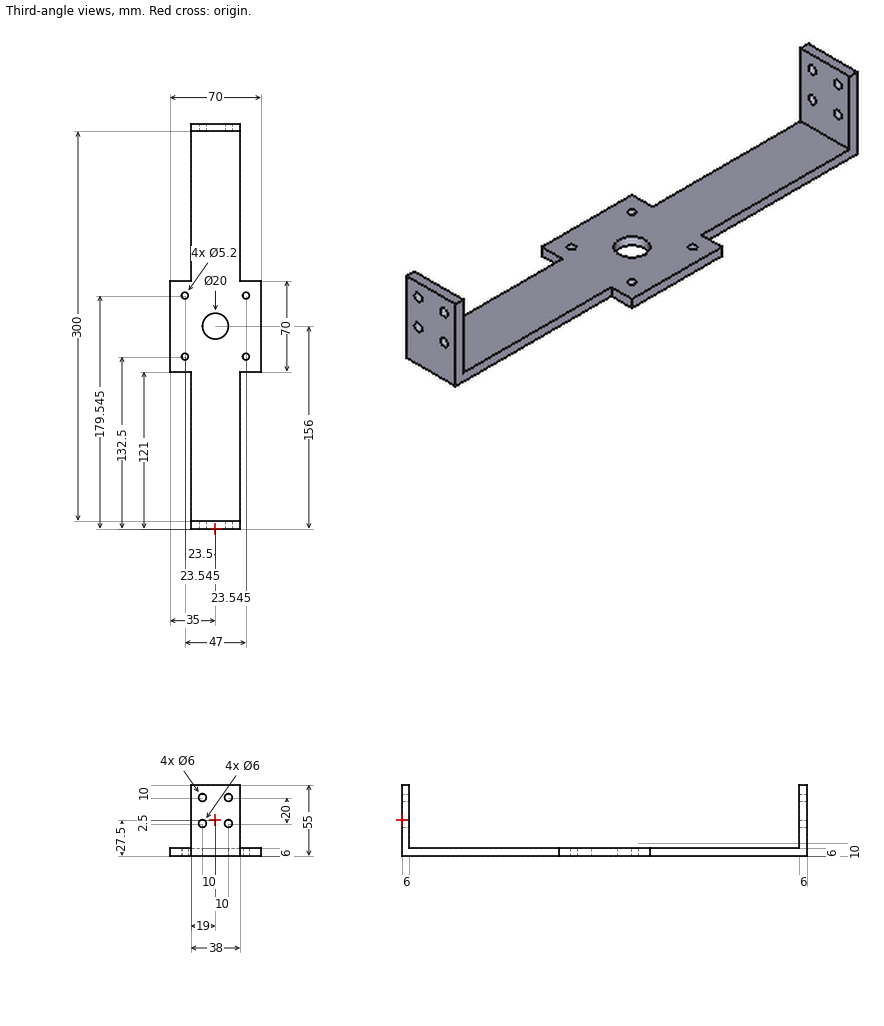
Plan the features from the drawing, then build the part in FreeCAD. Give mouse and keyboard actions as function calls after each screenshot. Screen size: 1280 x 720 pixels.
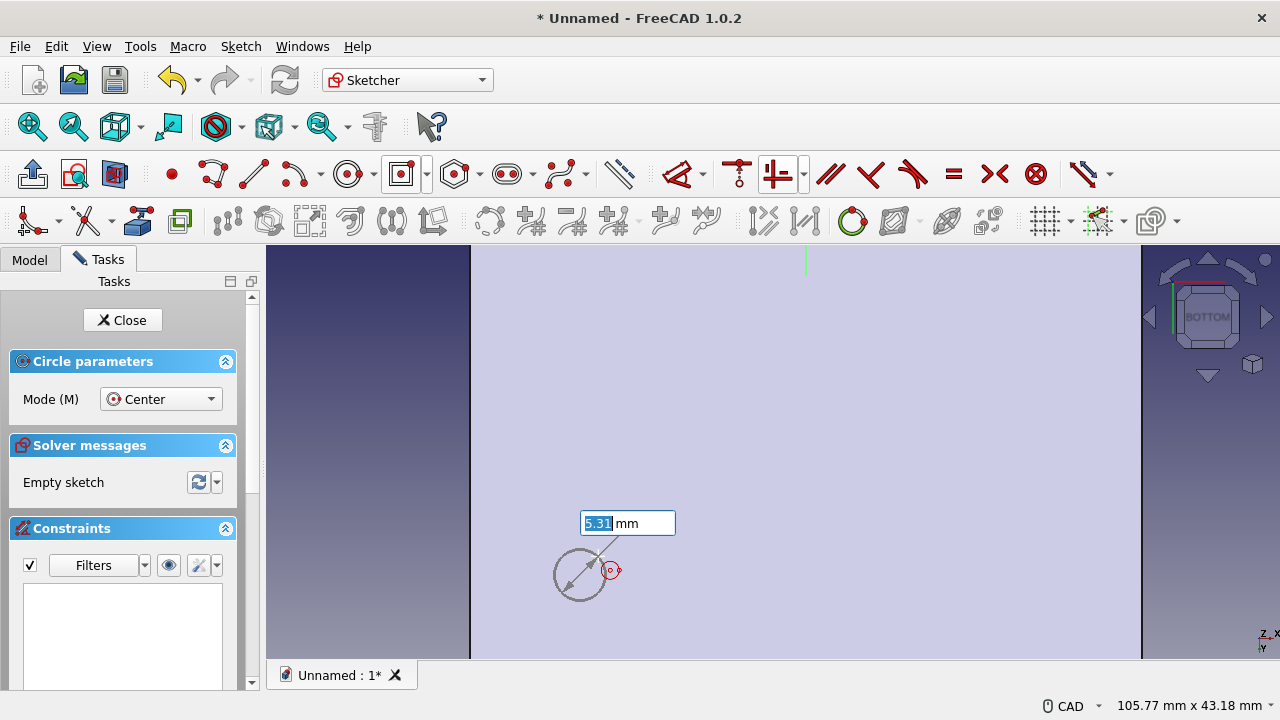
text(5.2)
key(Return)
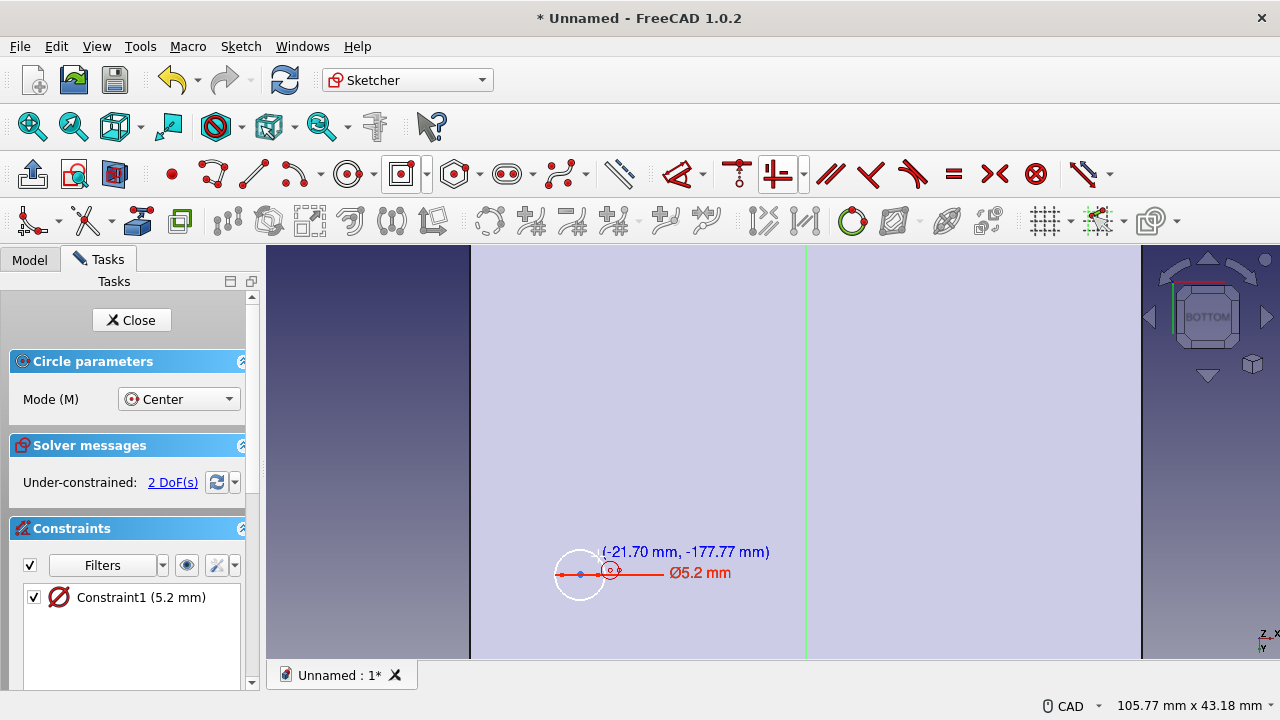
scroll(581, 578, down, 3)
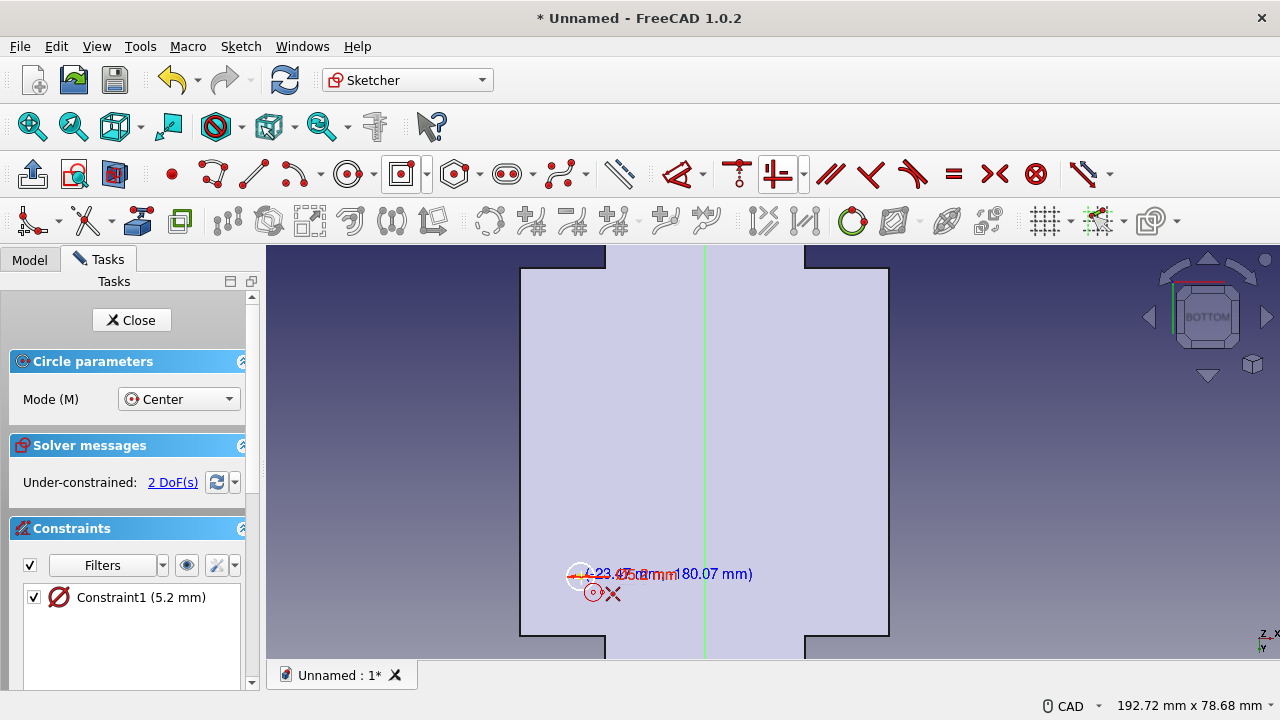
scroll(581, 329, up, 3)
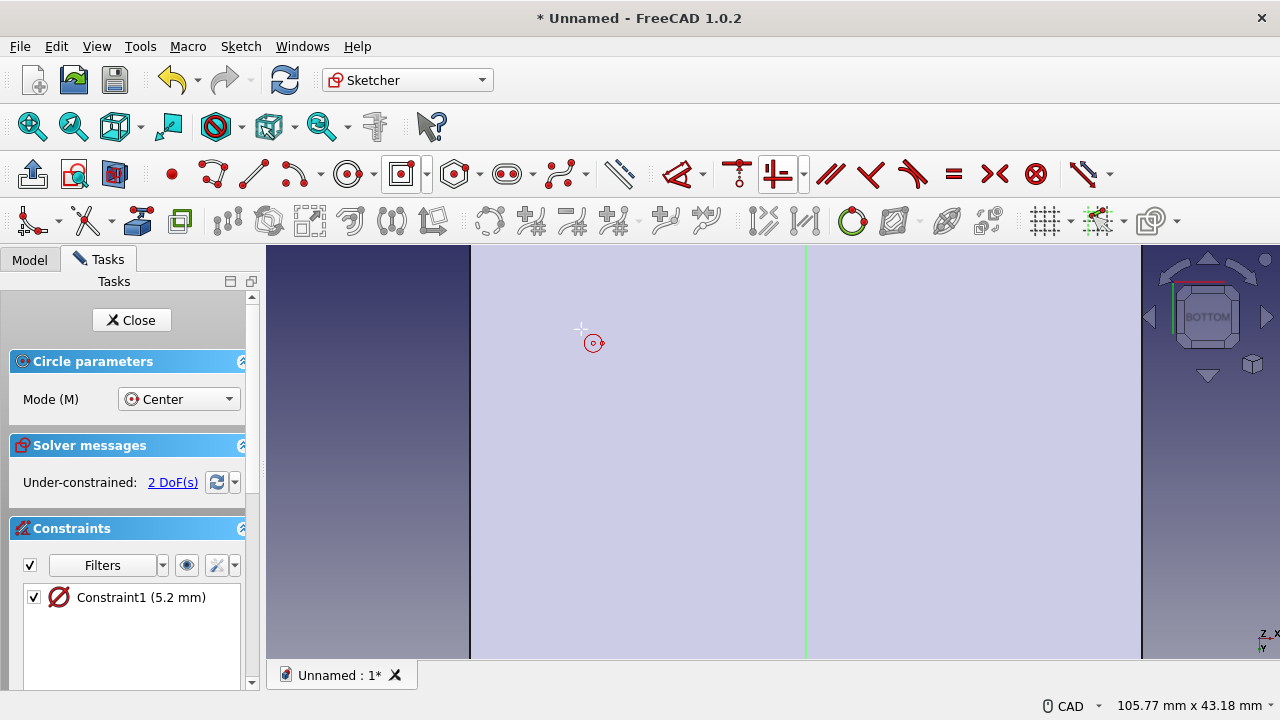
click(581, 328)
move(598, 311)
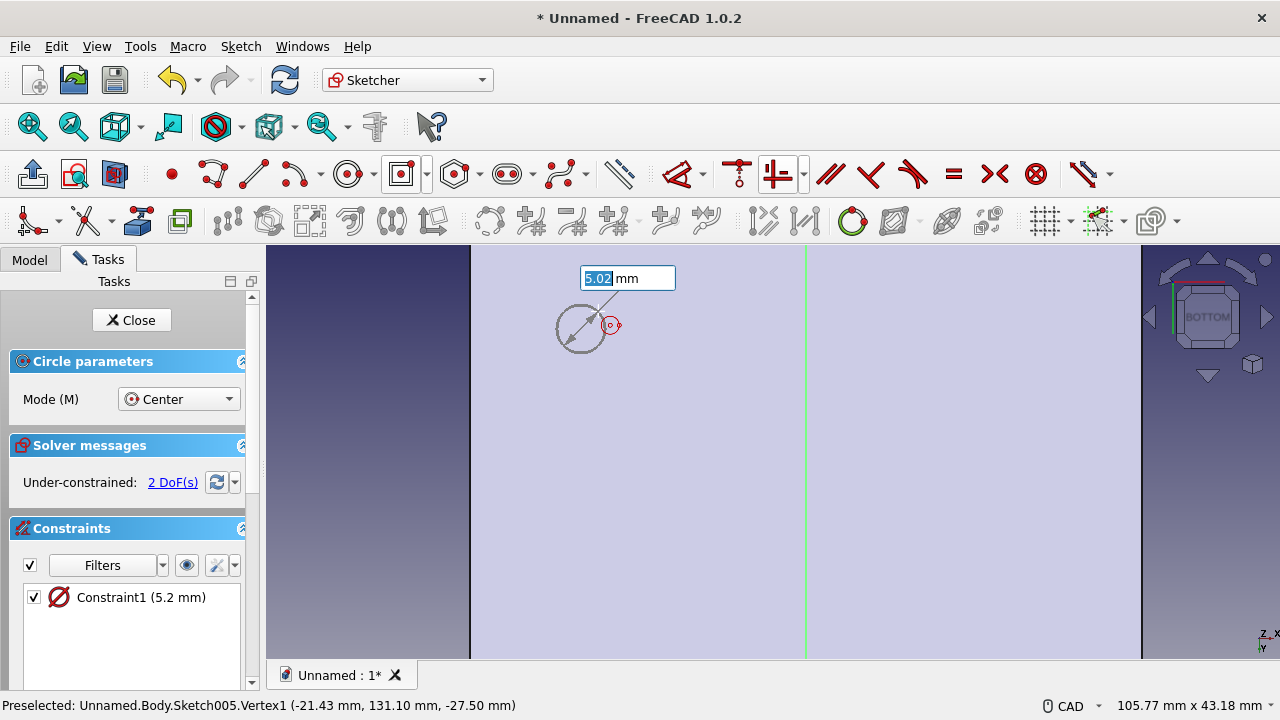
text(5.2)
key(Return)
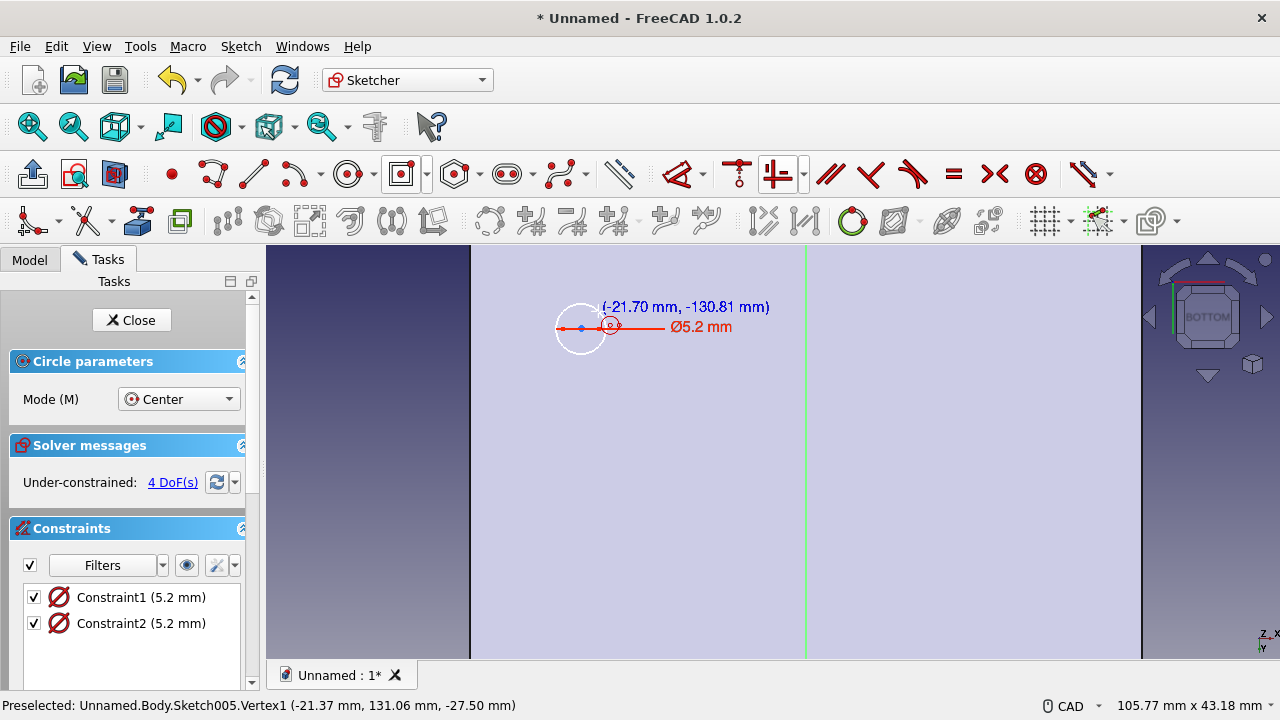
click(1031, 328)
move(1049, 311)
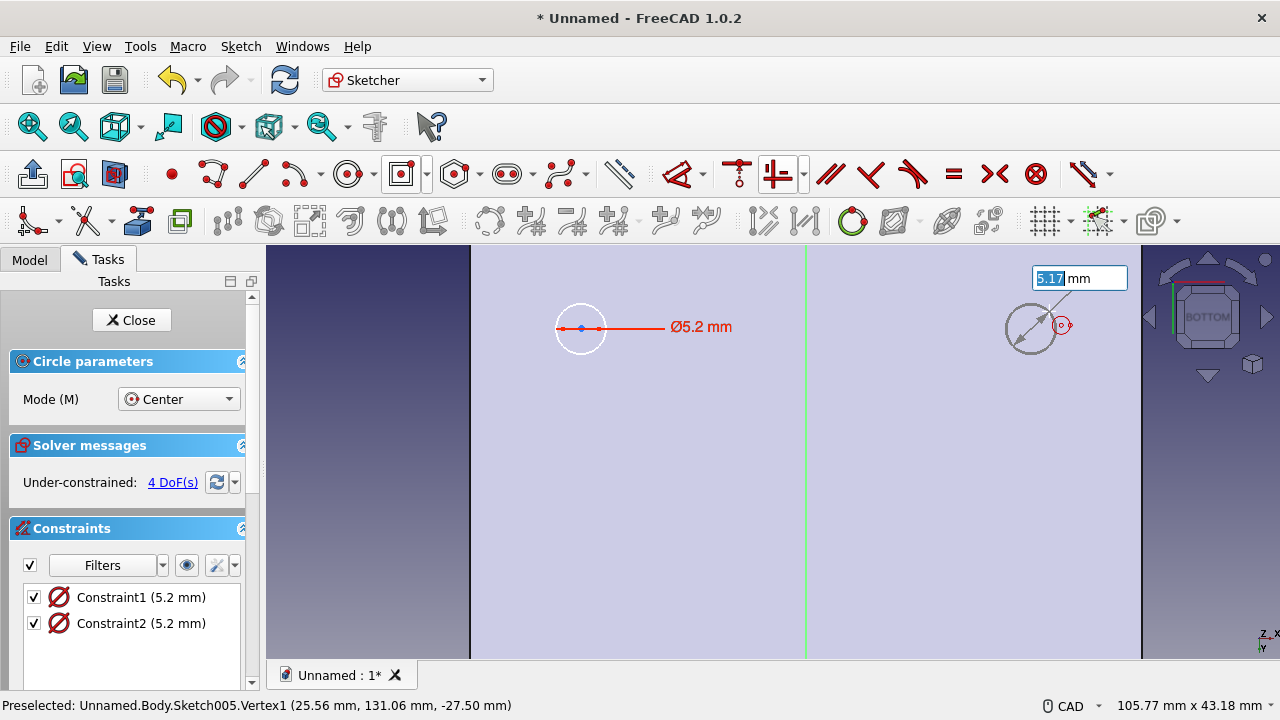
text(5.2)
key(Return)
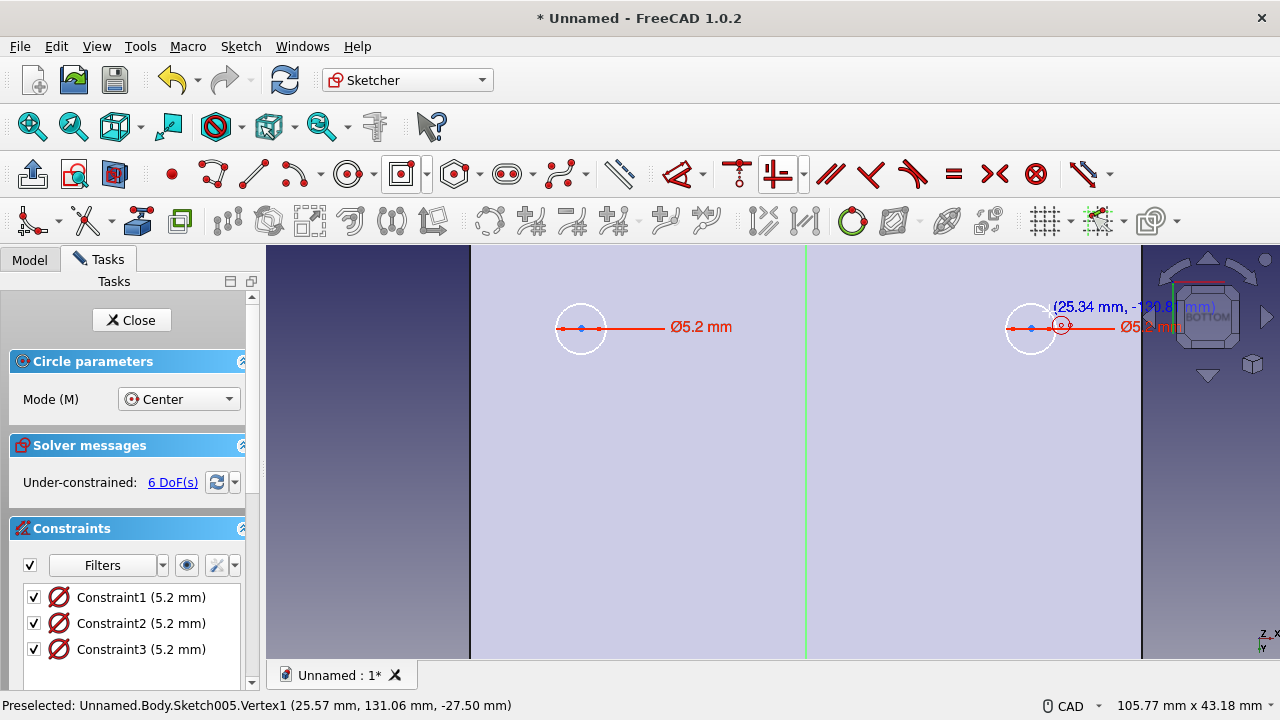
scroll(581, 328, down, 3)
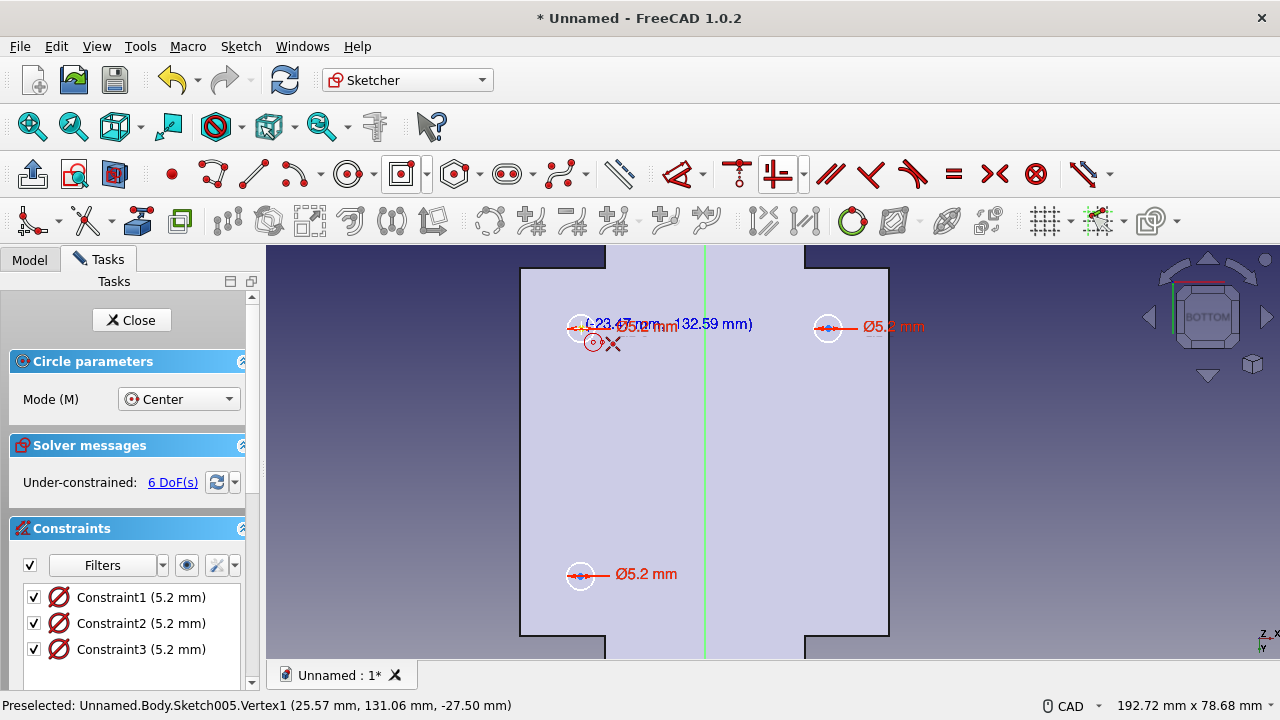
scroll(829, 576, up, 3)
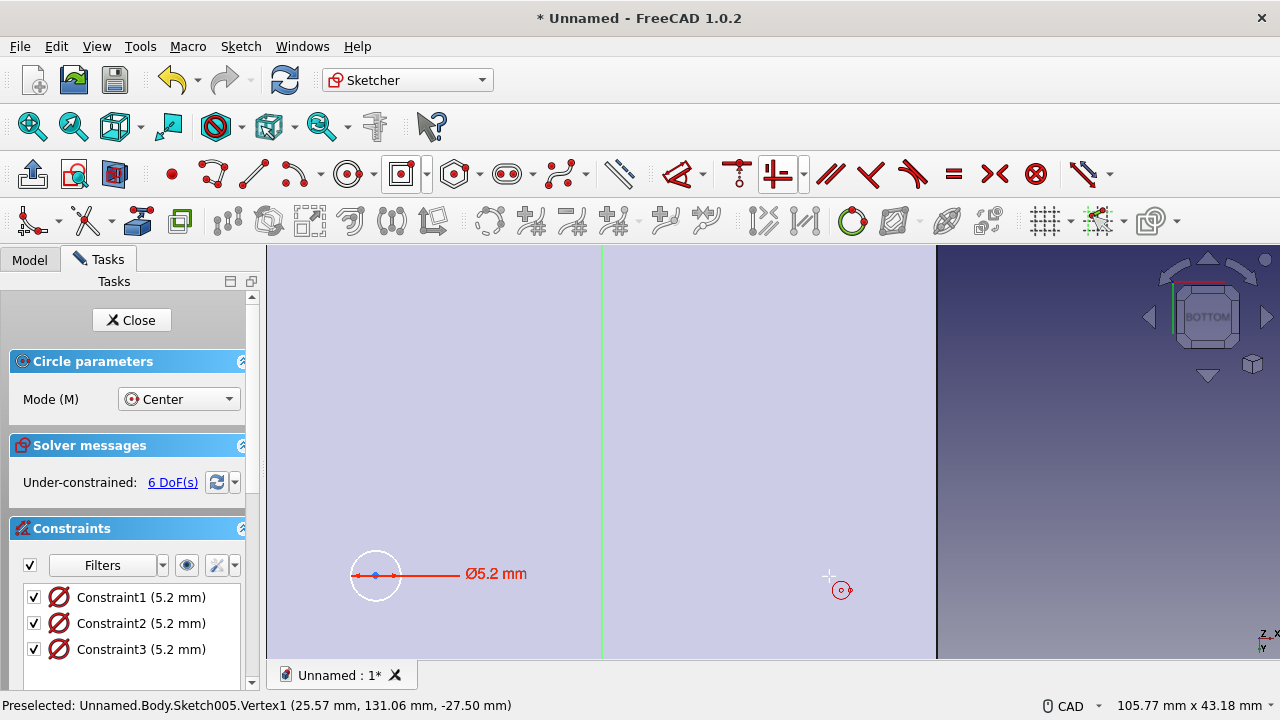
click(828, 575)
move(845, 557)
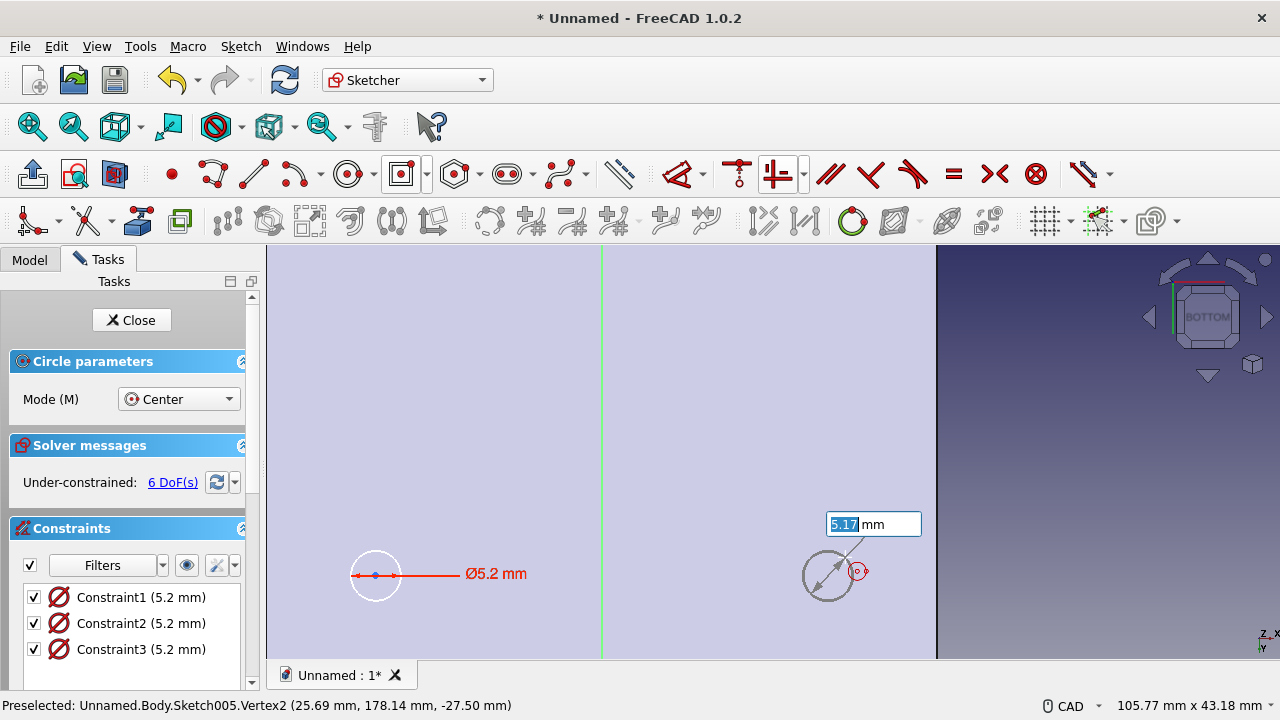
text(5.2)
key(Return)